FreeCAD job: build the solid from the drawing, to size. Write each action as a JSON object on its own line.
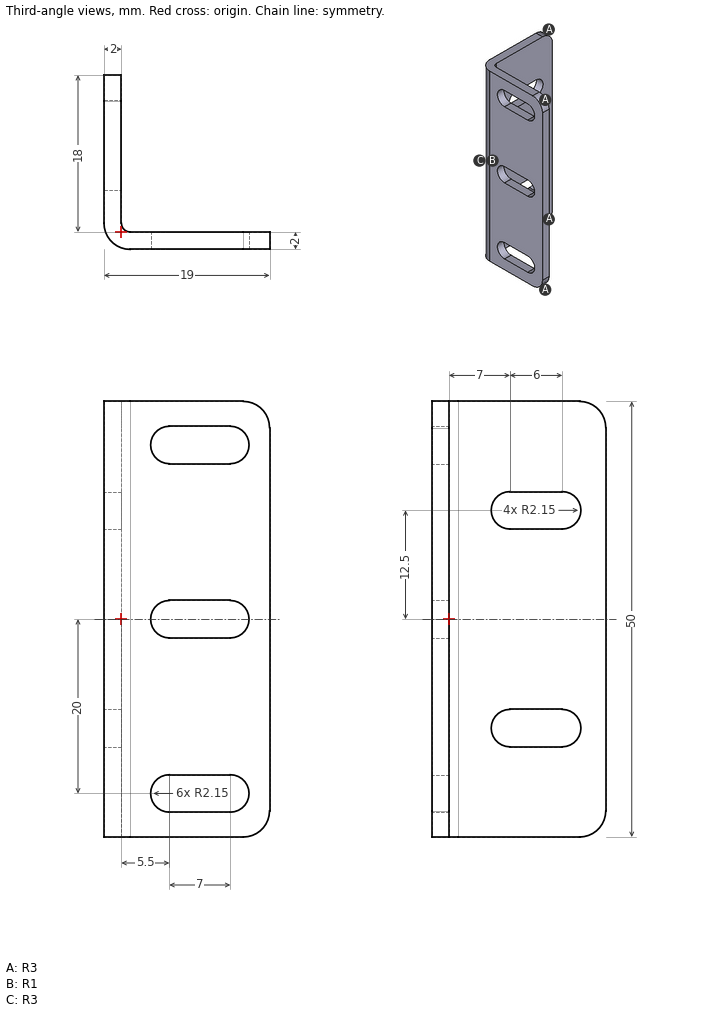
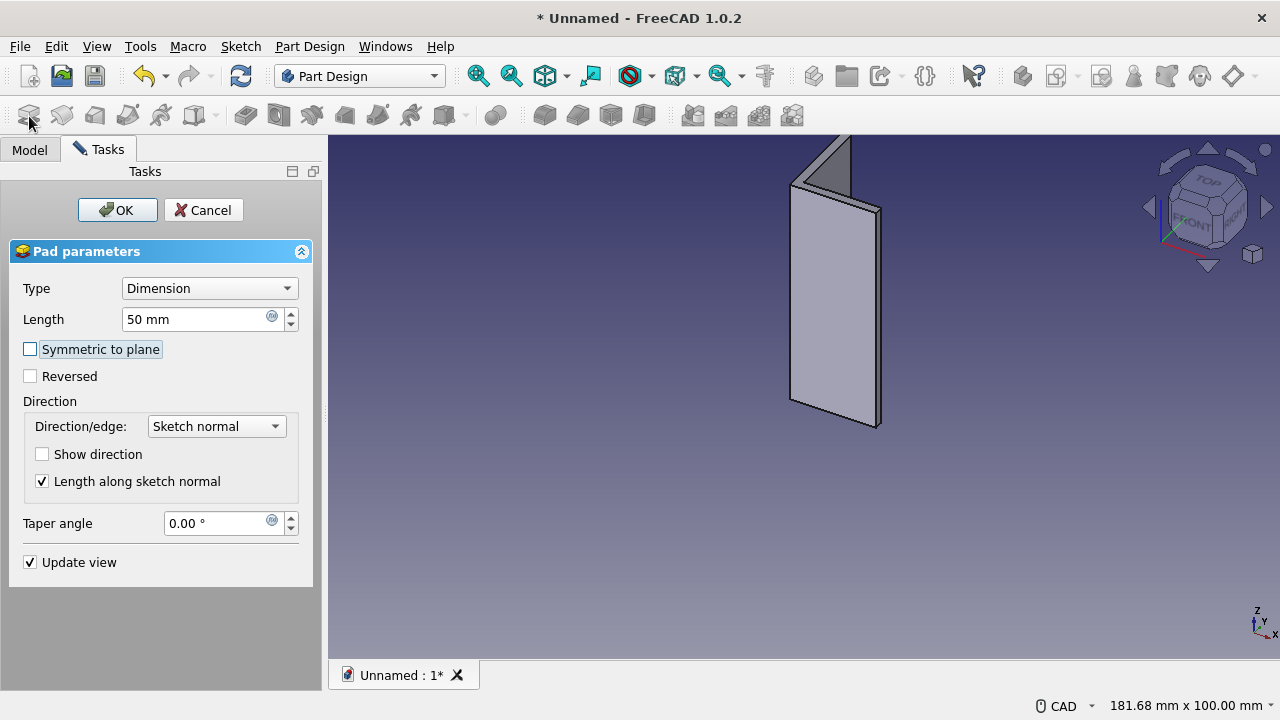
{"action": "left_click", "coordinate": [31, 349]}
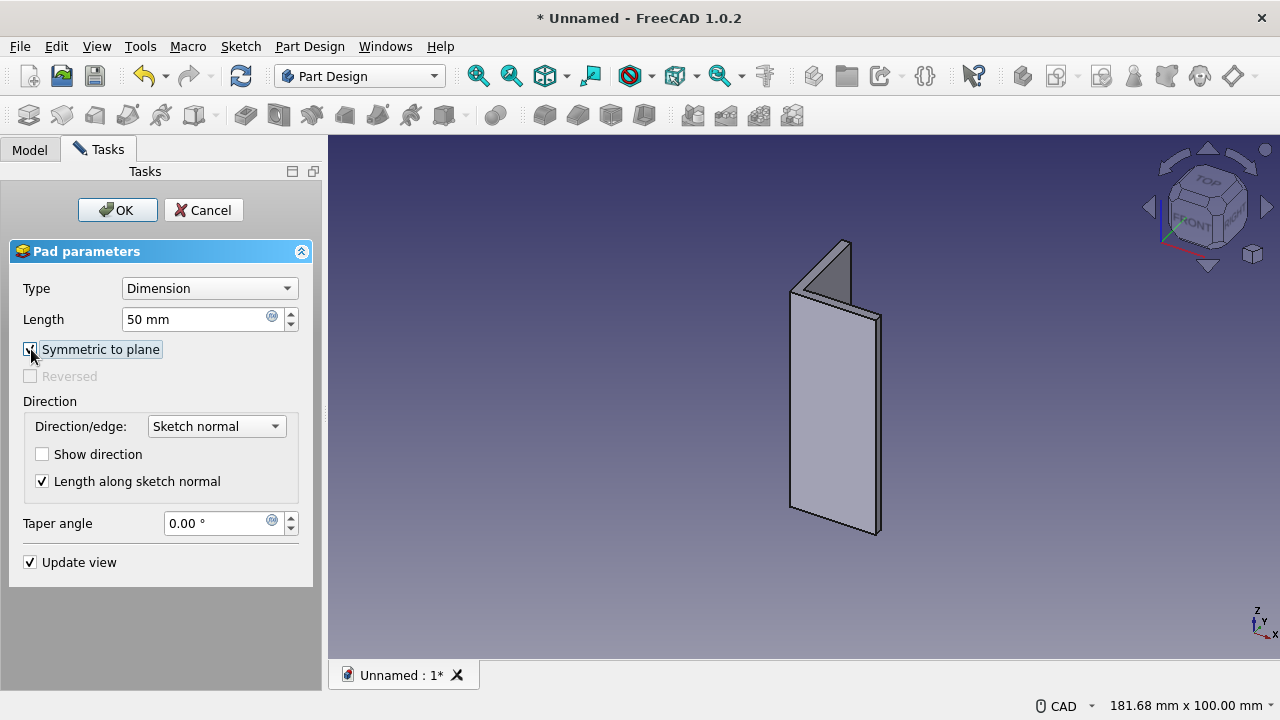
{"action": "left_click", "coordinate": [118, 210]}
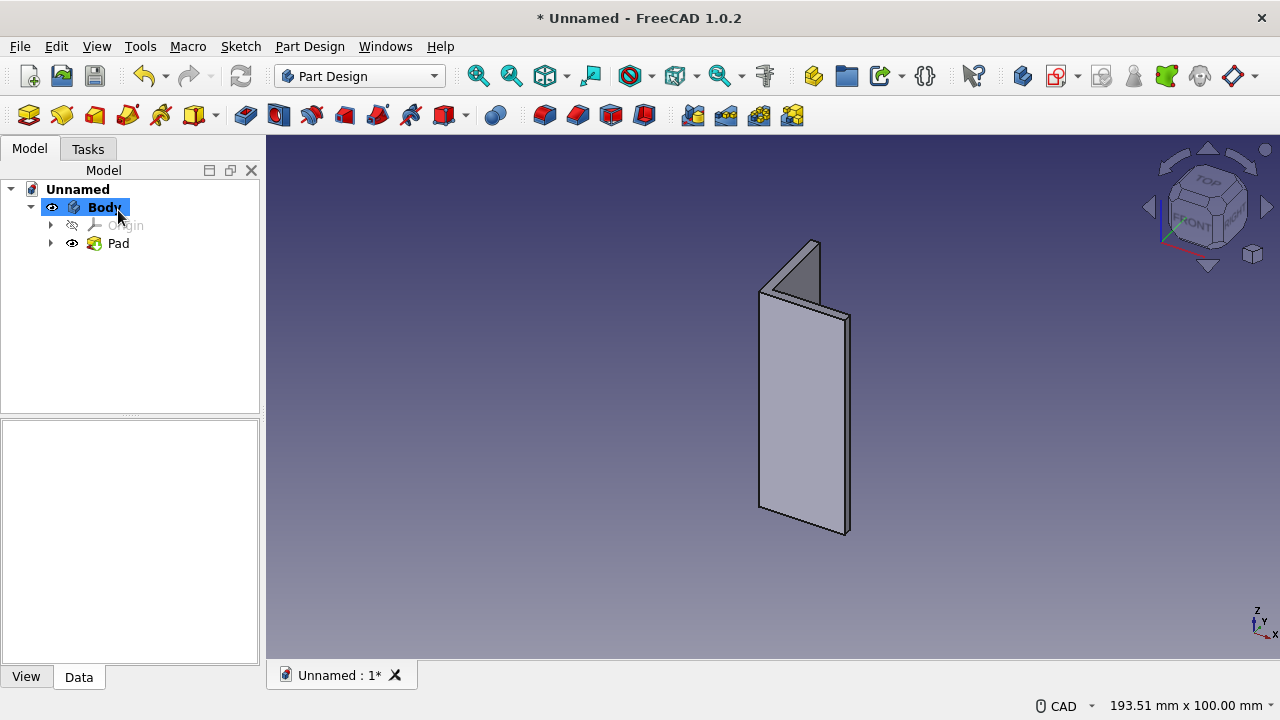
{"action": "left_click", "coordinate": [1056, 76]}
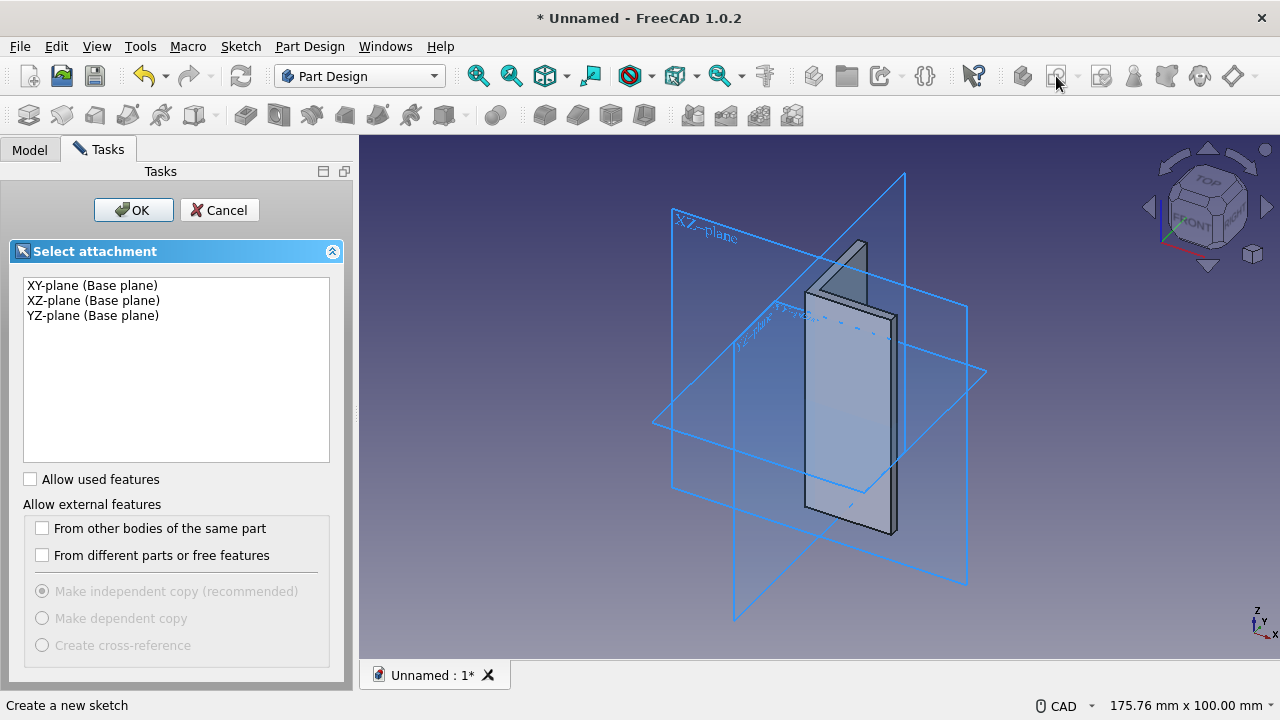
{"action": "left_click", "coordinate": [84, 300]}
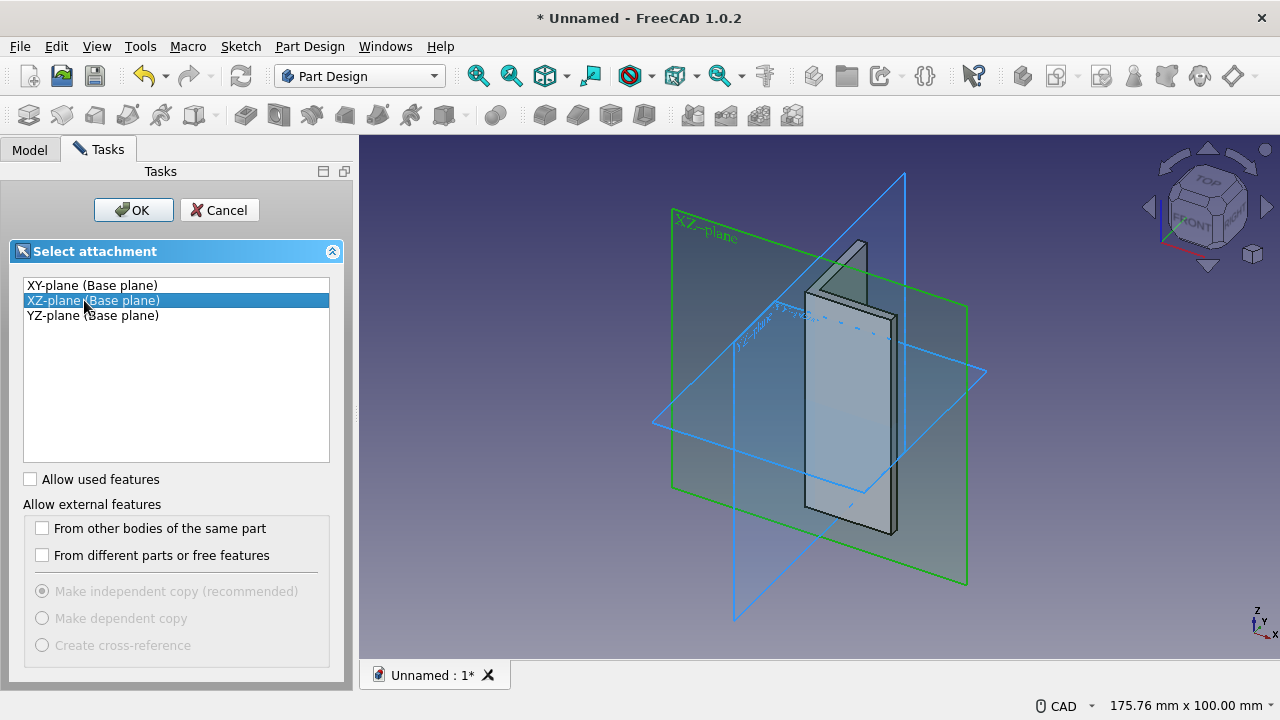
{"action": "left_click", "coordinate": [134, 210]}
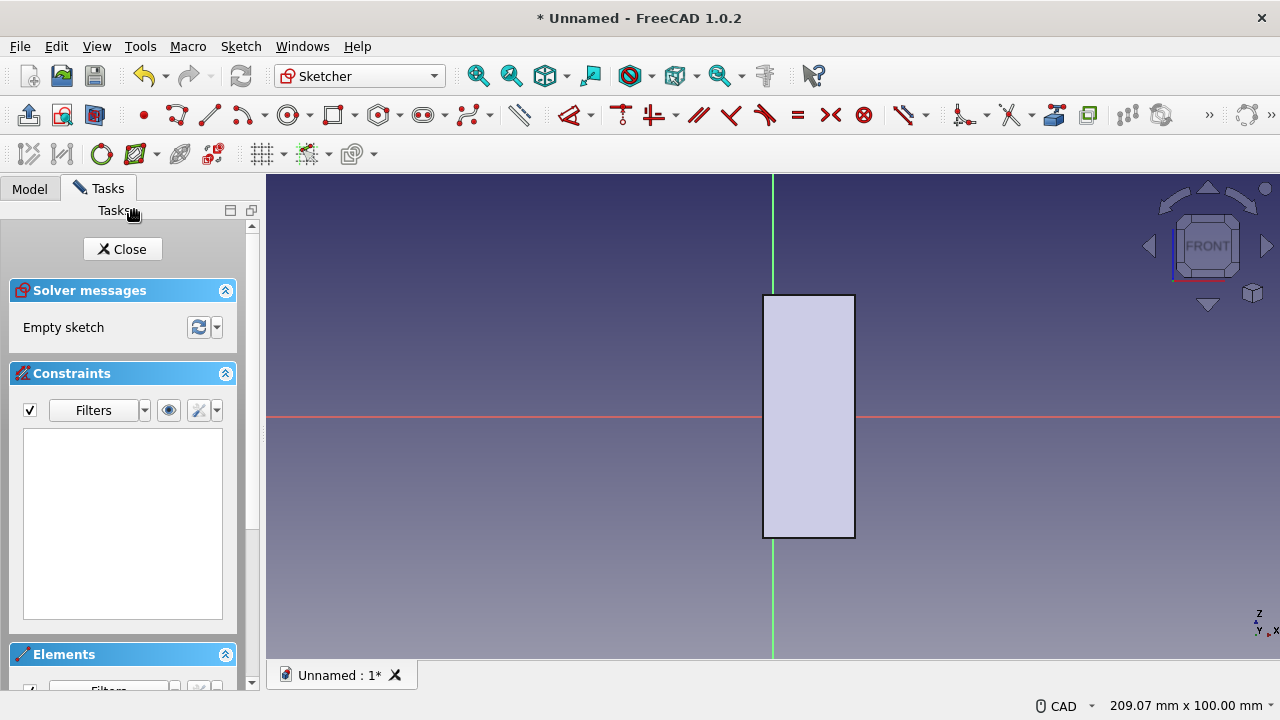
{"action": "left_click", "coordinate": [95, 116]}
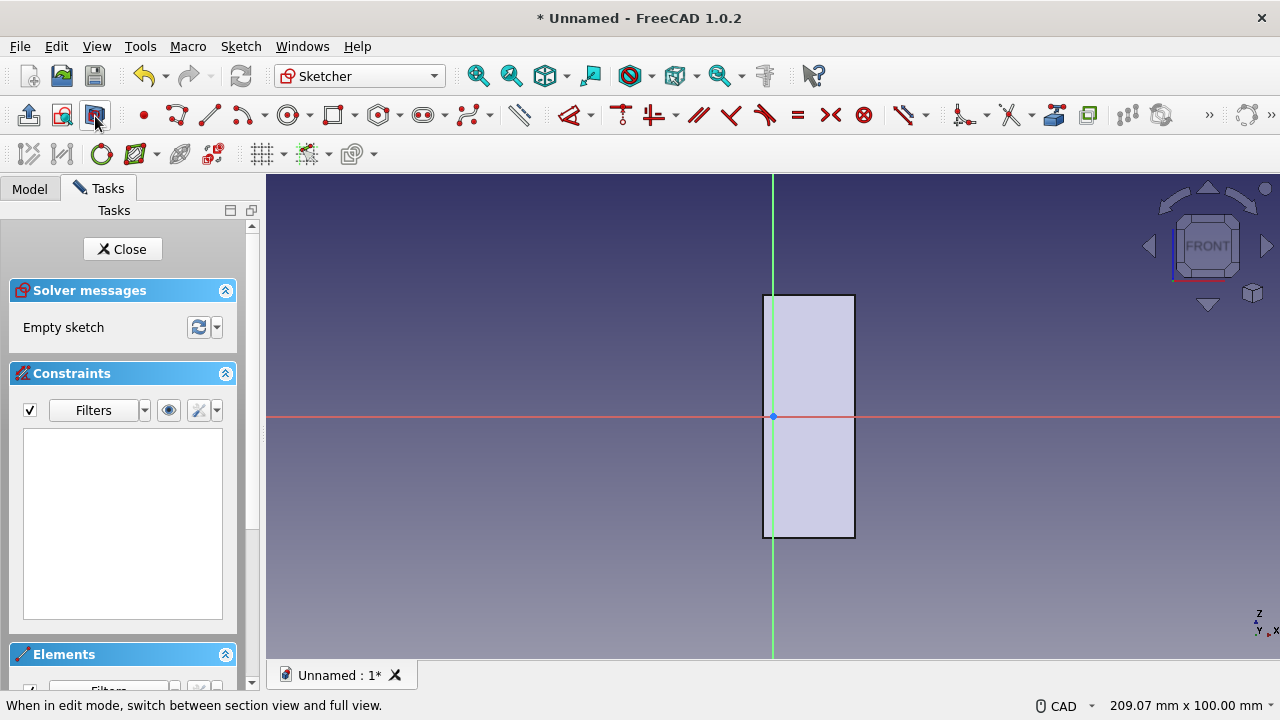
{"action": "scroll", "coordinate": [1020, 416], "scroll_direction": "up", "scroll_amount": 2}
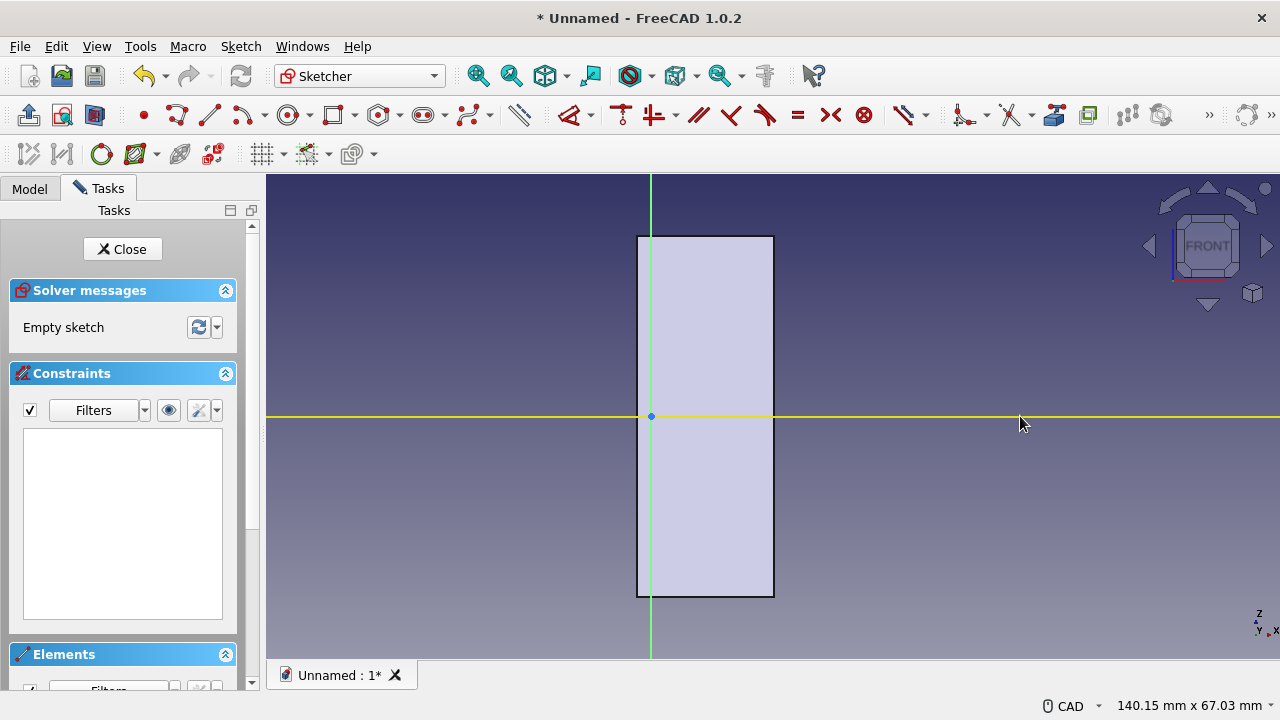
{"action": "left_click", "coordinate": [422, 116]}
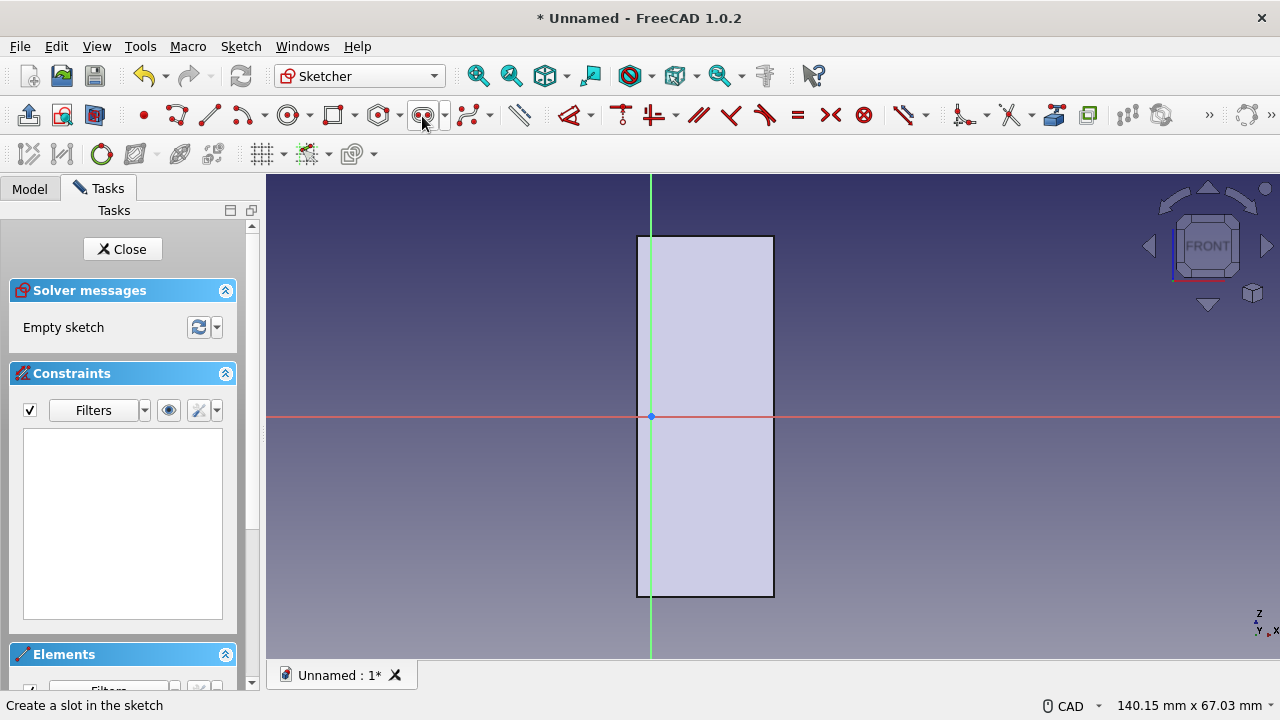
{"action": "scroll", "coordinate": [691, 561], "scroll_direction": "up", "scroll_amount": 2}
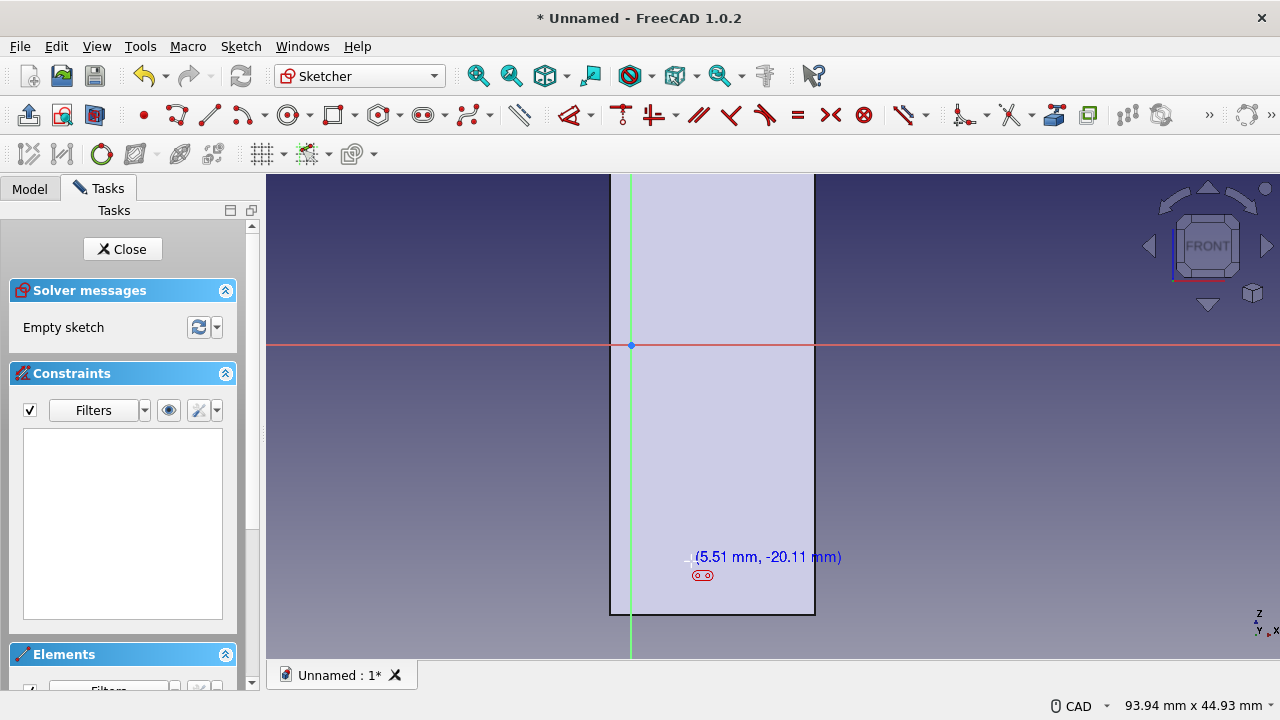
{"action": "left_click", "coordinate": [691, 561]}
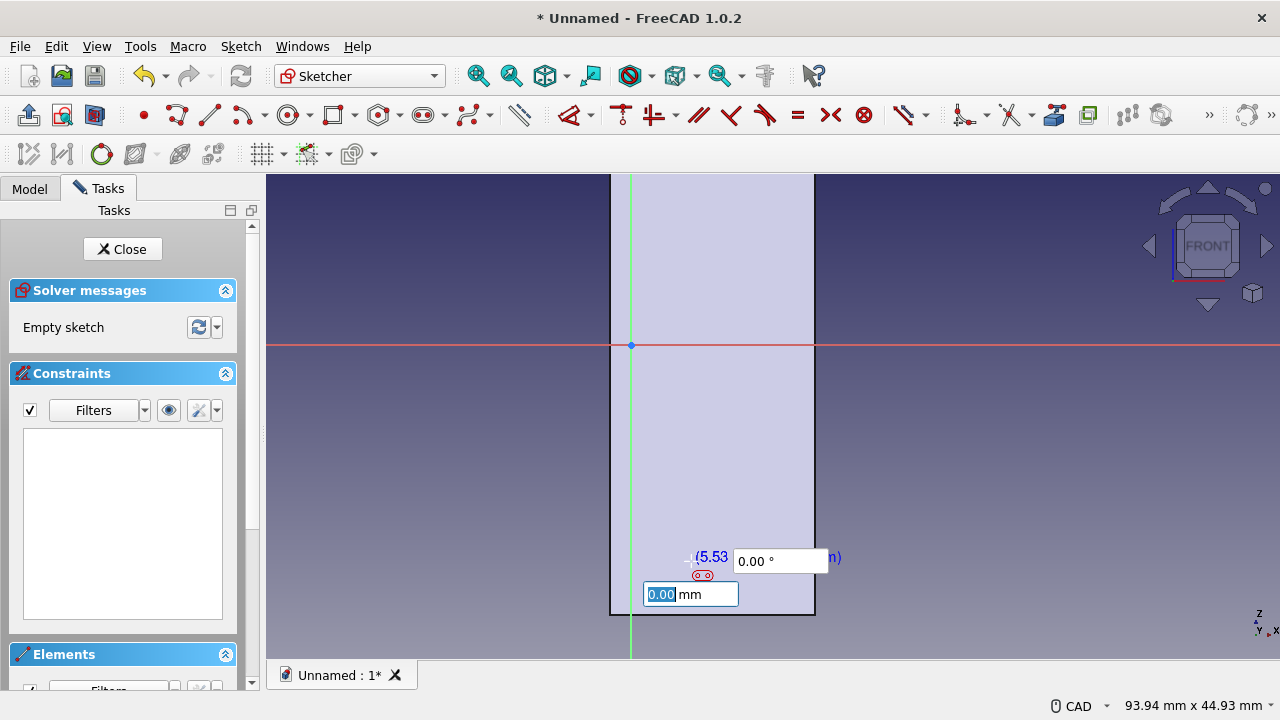
{"action": "left_click", "coordinate": [766, 561]}